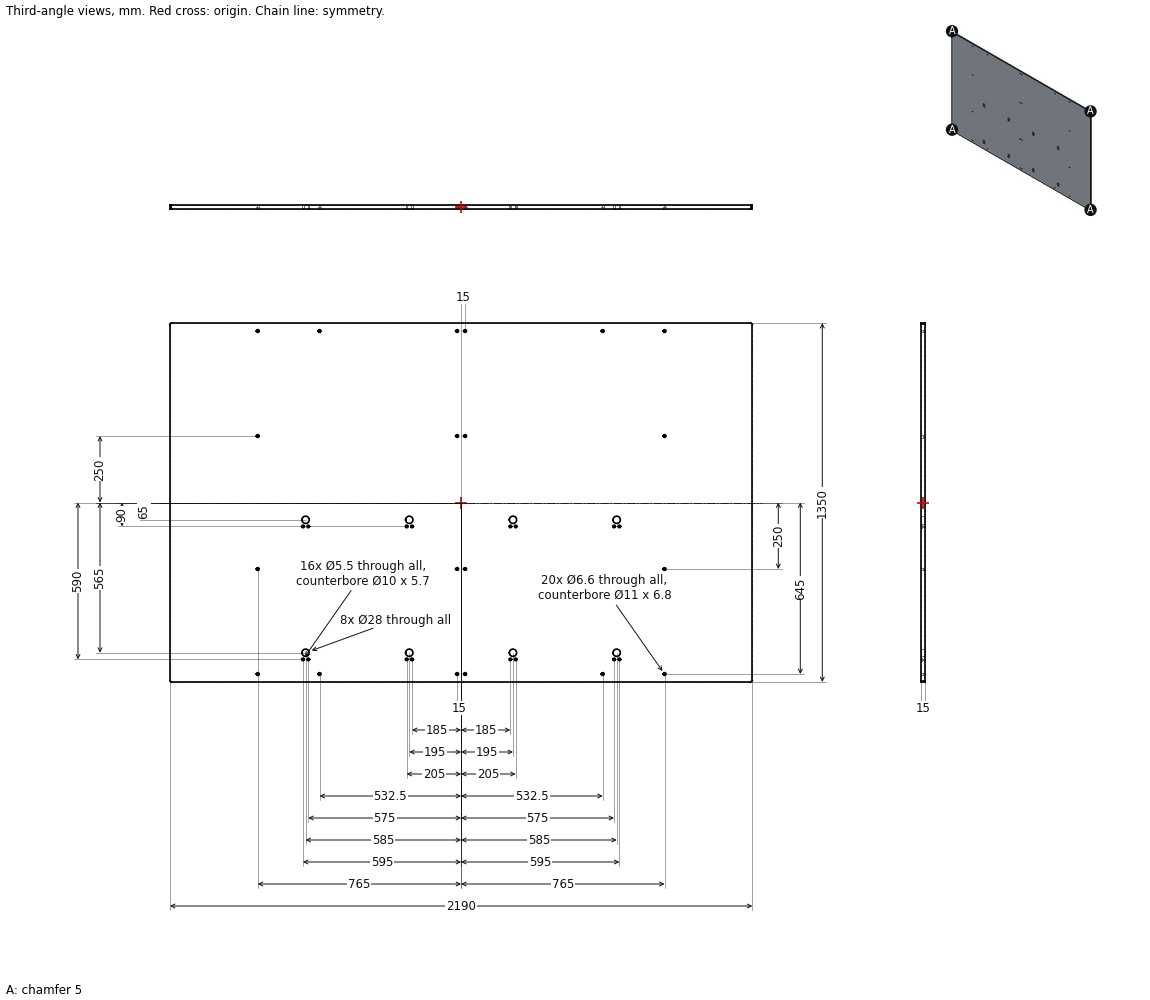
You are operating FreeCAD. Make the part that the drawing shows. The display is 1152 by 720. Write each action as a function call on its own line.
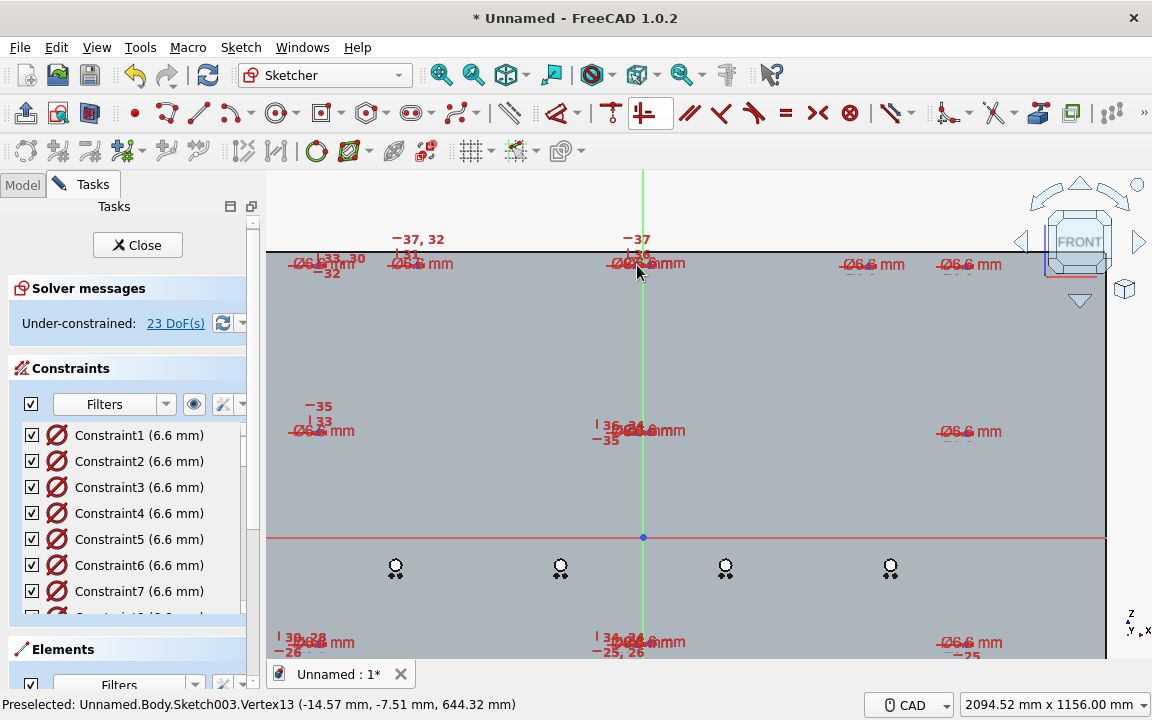
scroll(637, 265, down, 3)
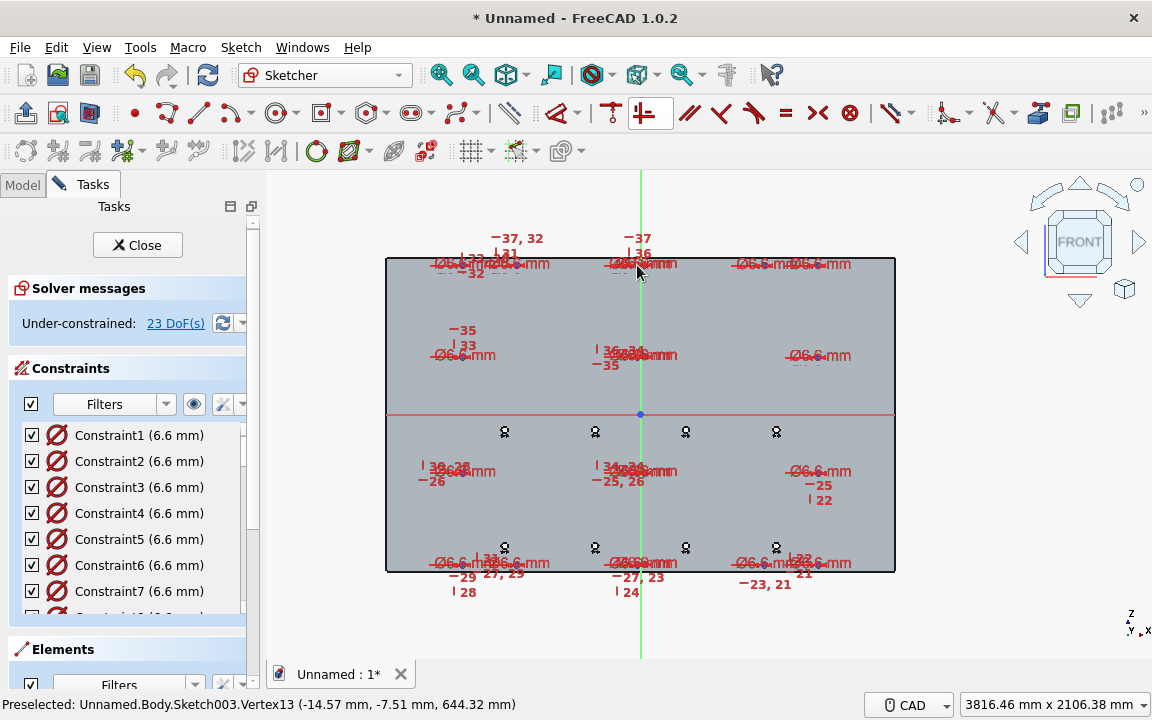
click(818, 473)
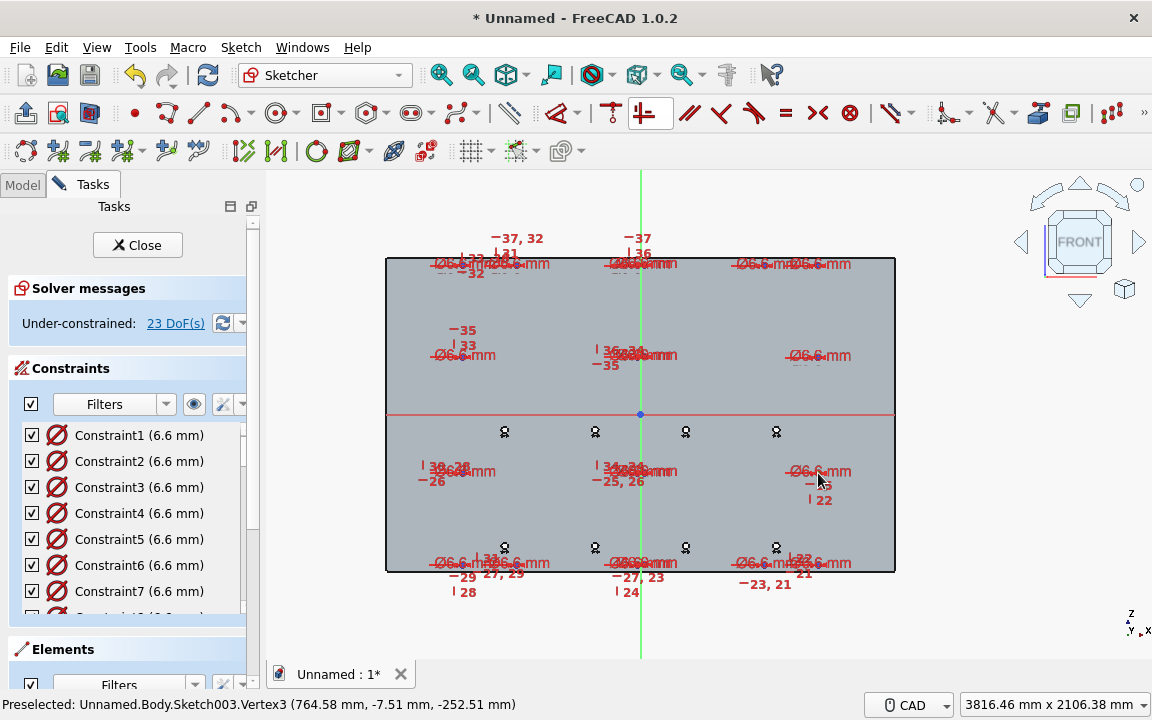
click(818, 358)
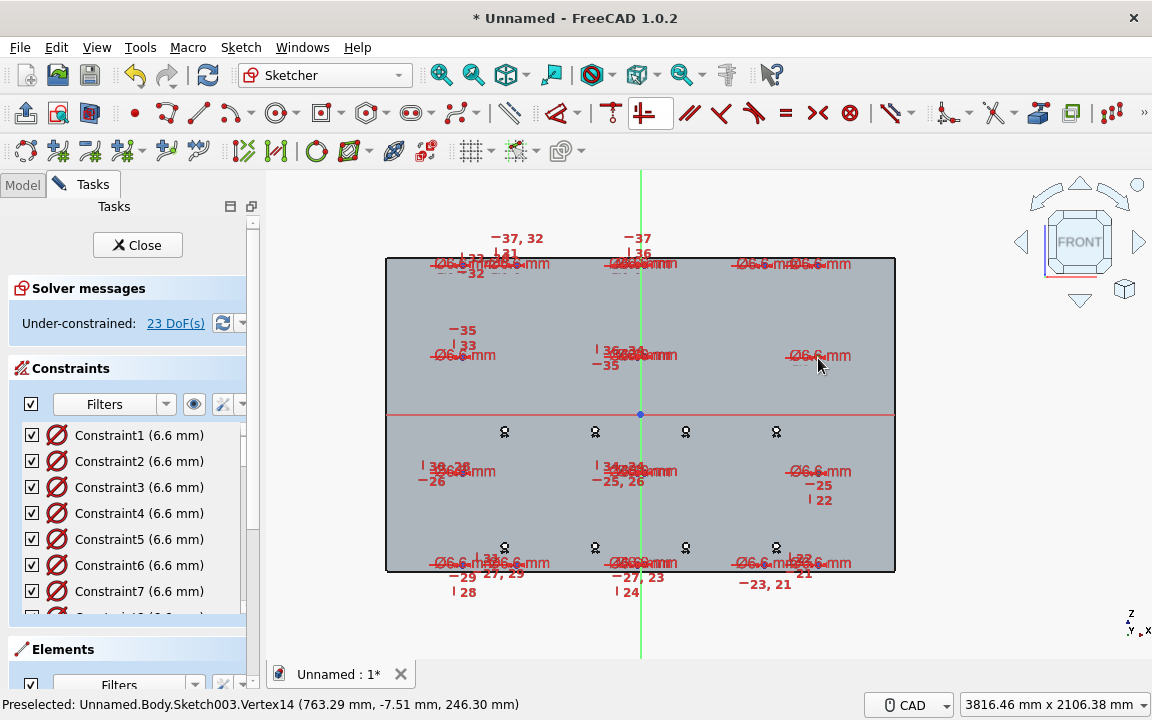
click(668, 114)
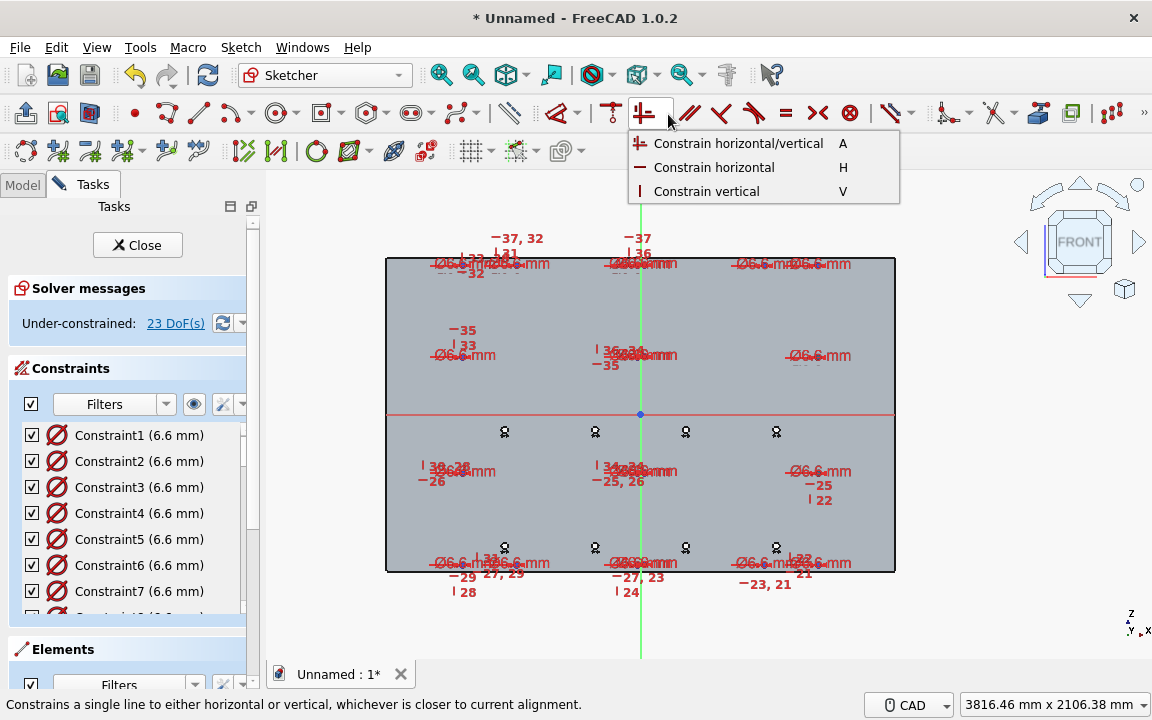
click(764, 191)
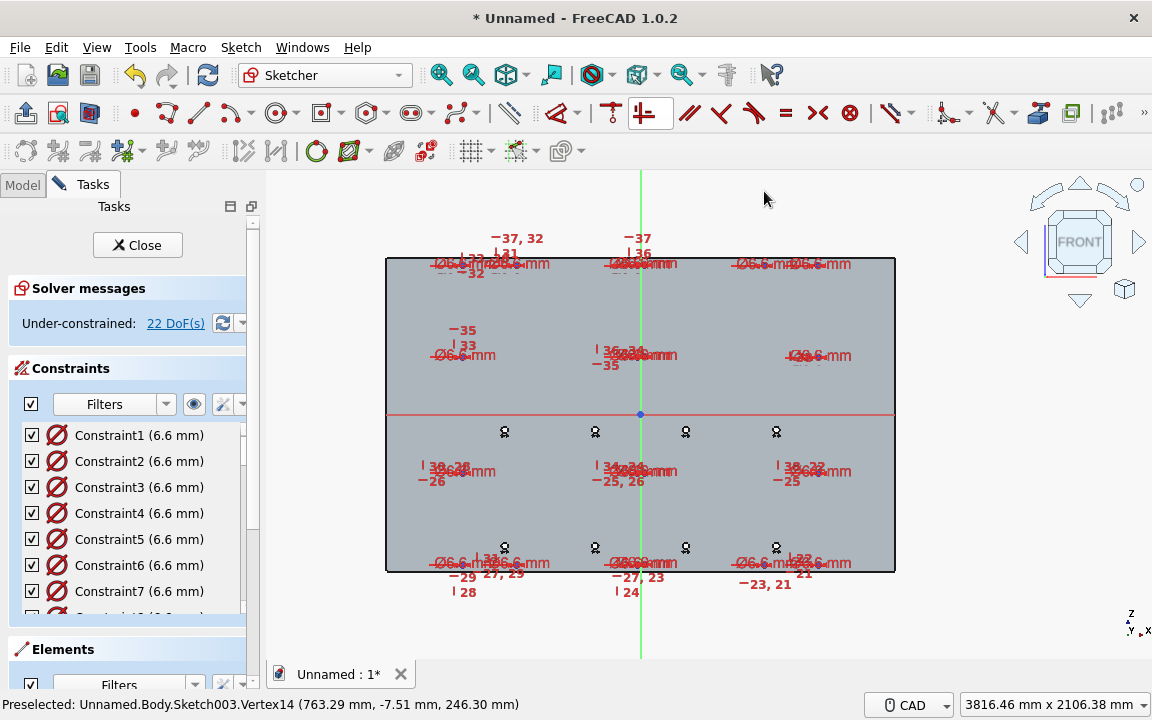
scroll(637, 357, up, 3)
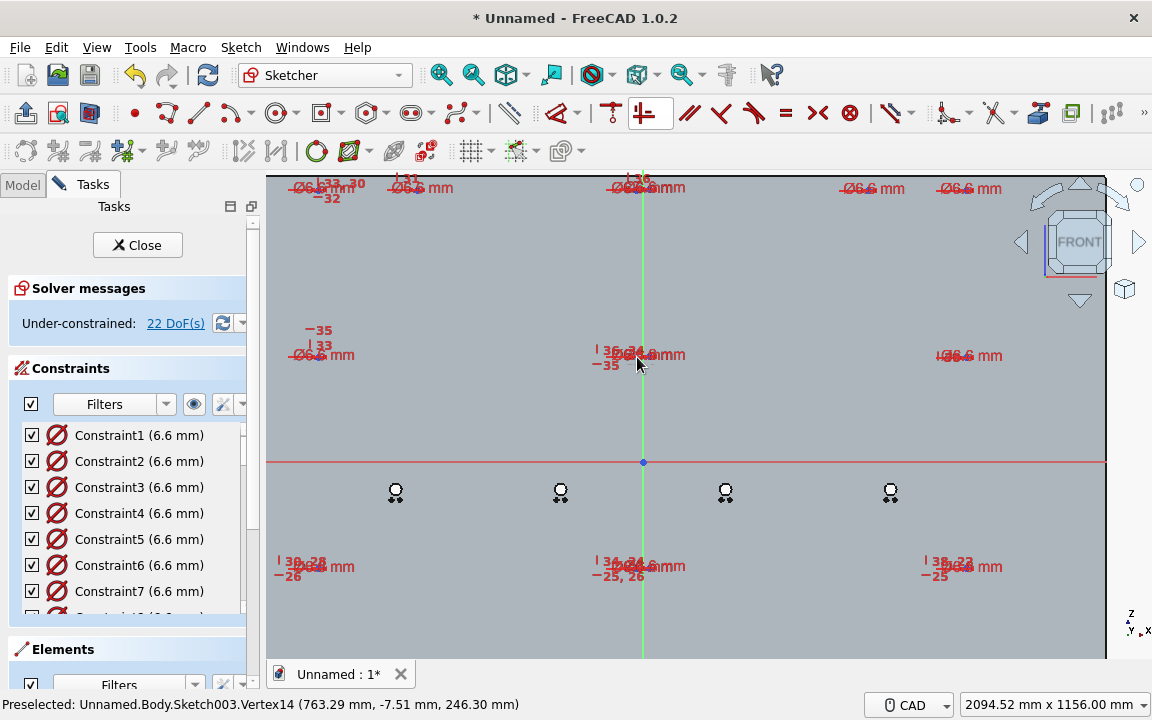
click(637, 357)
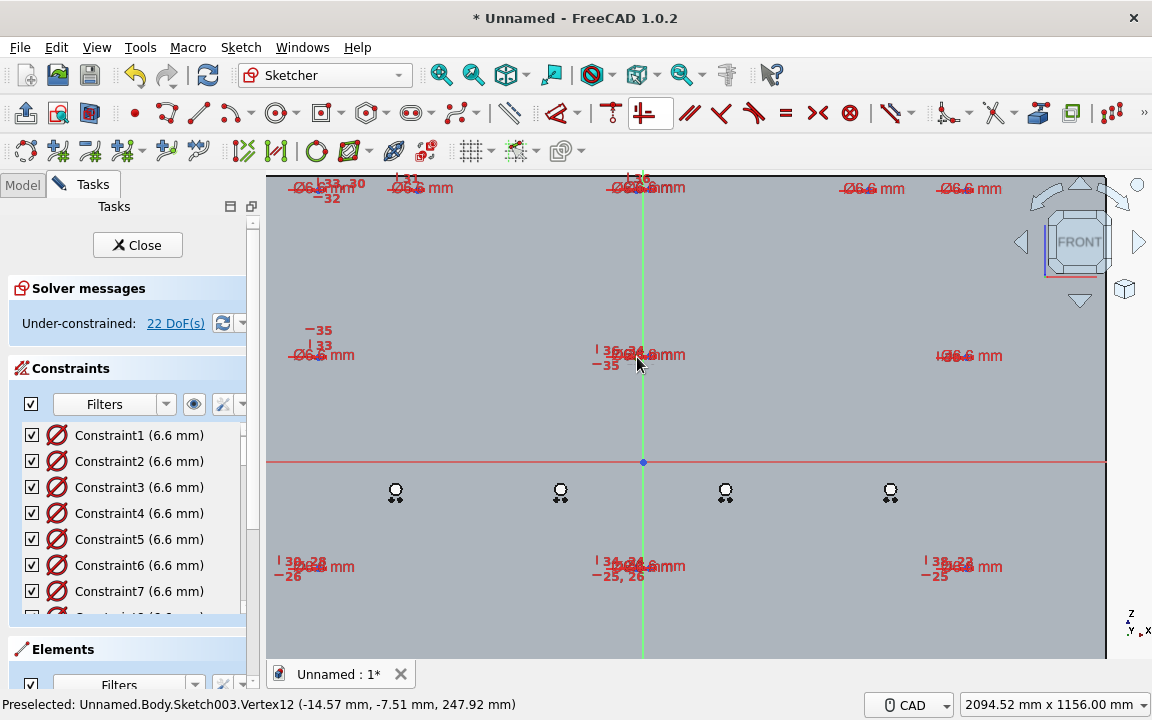
click(967, 358)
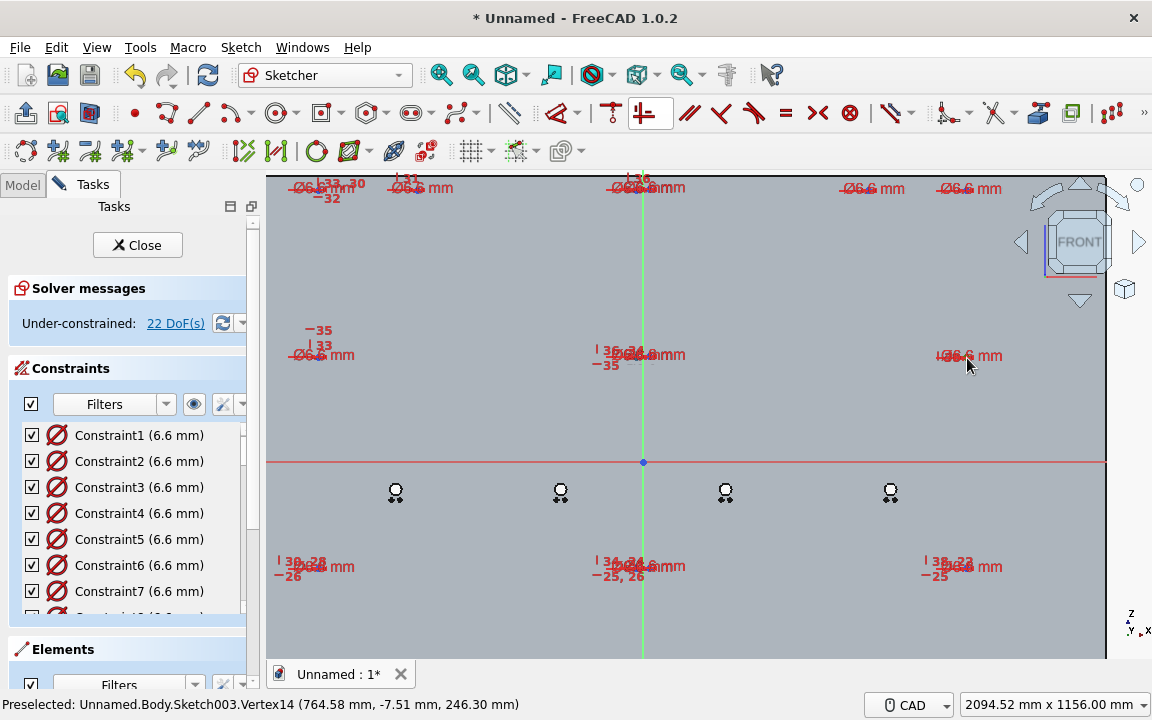
key(h)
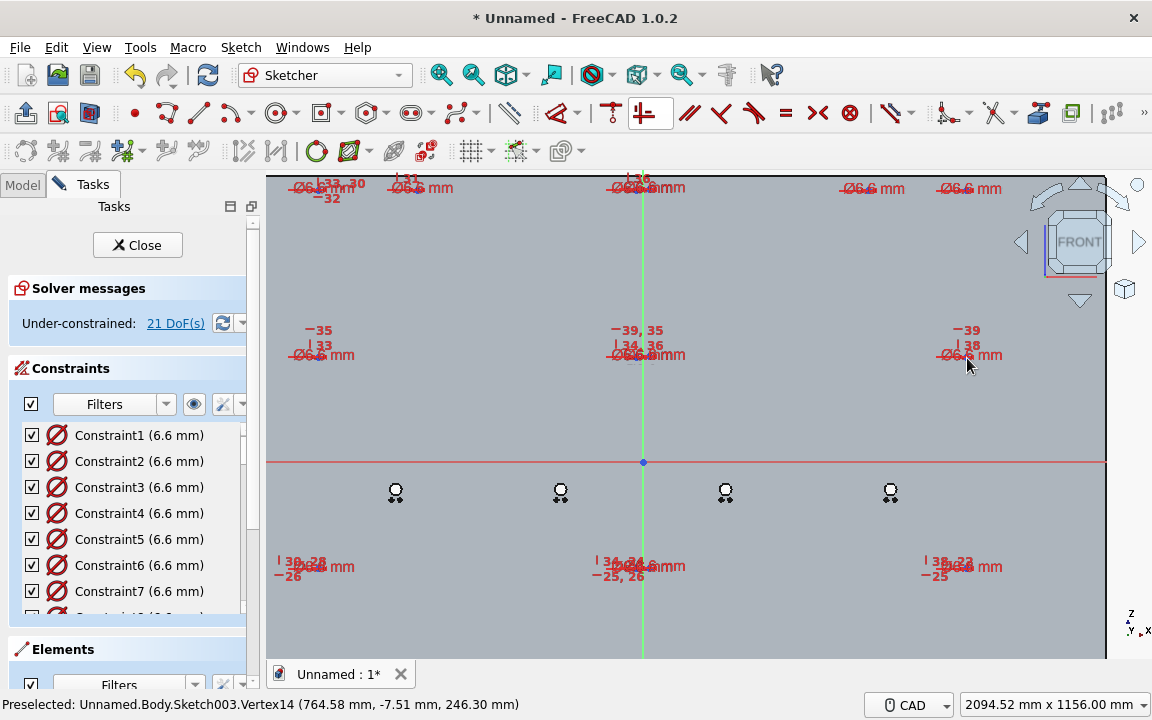
scroll(637, 357, down, 3)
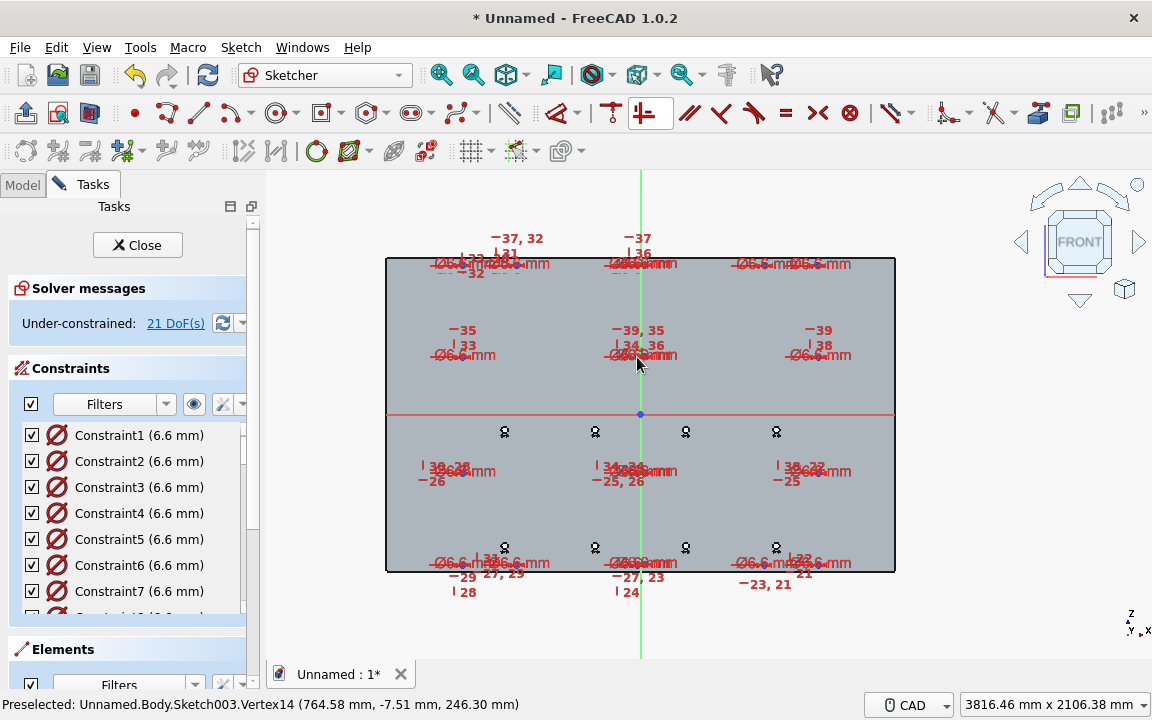
scroll(637, 266, up, 3)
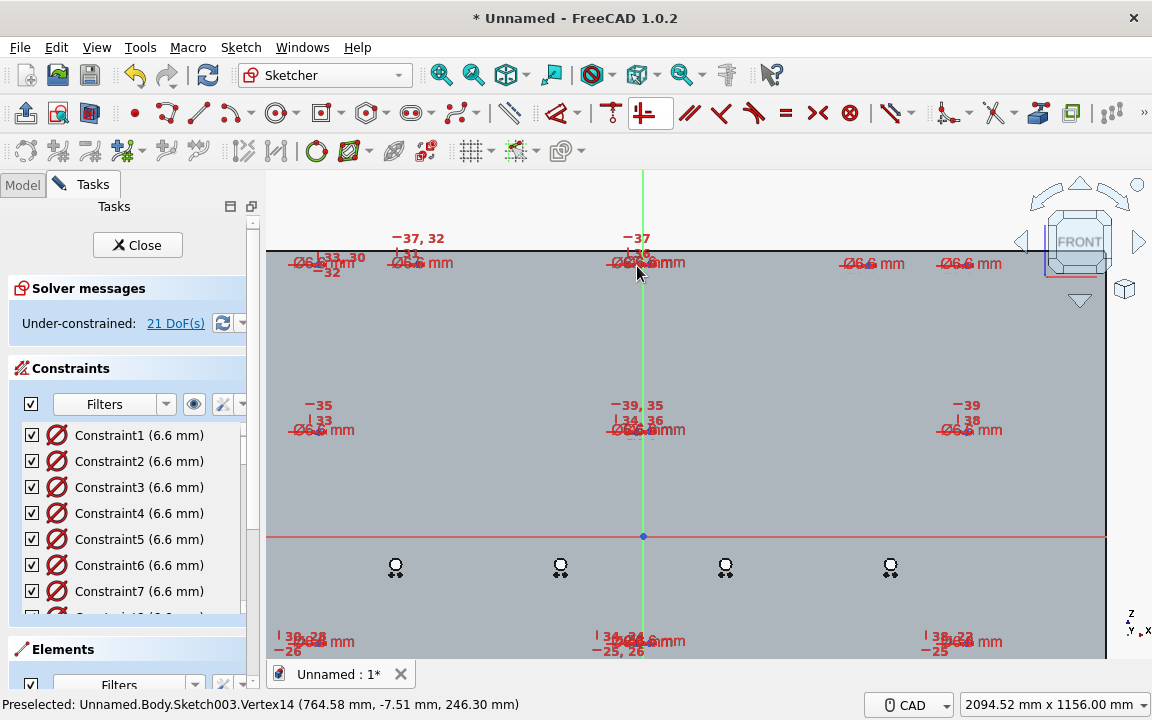
click(637, 265)